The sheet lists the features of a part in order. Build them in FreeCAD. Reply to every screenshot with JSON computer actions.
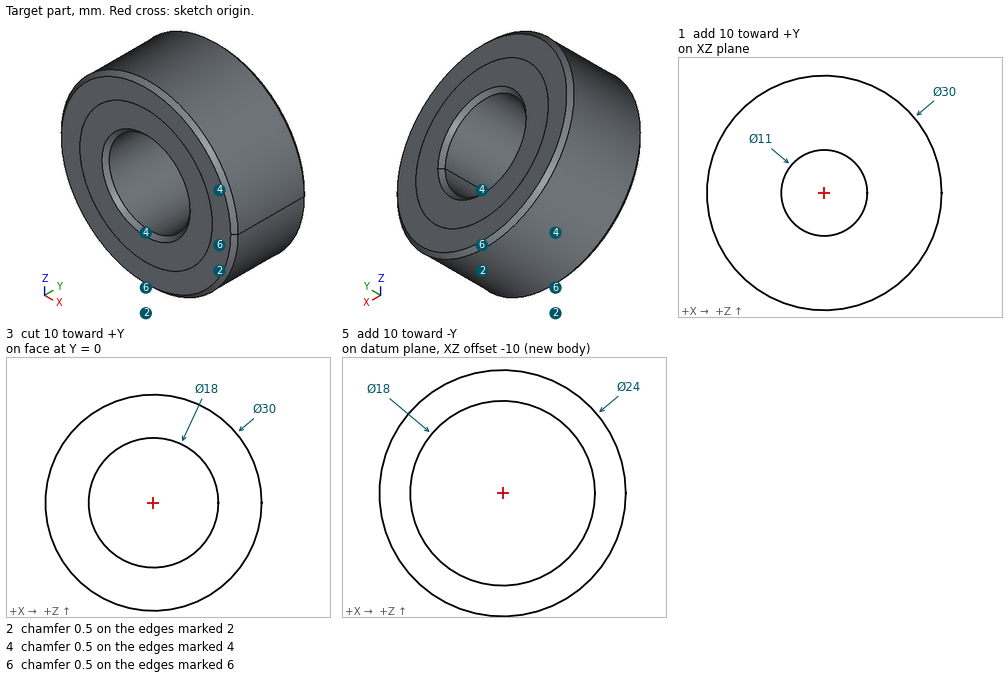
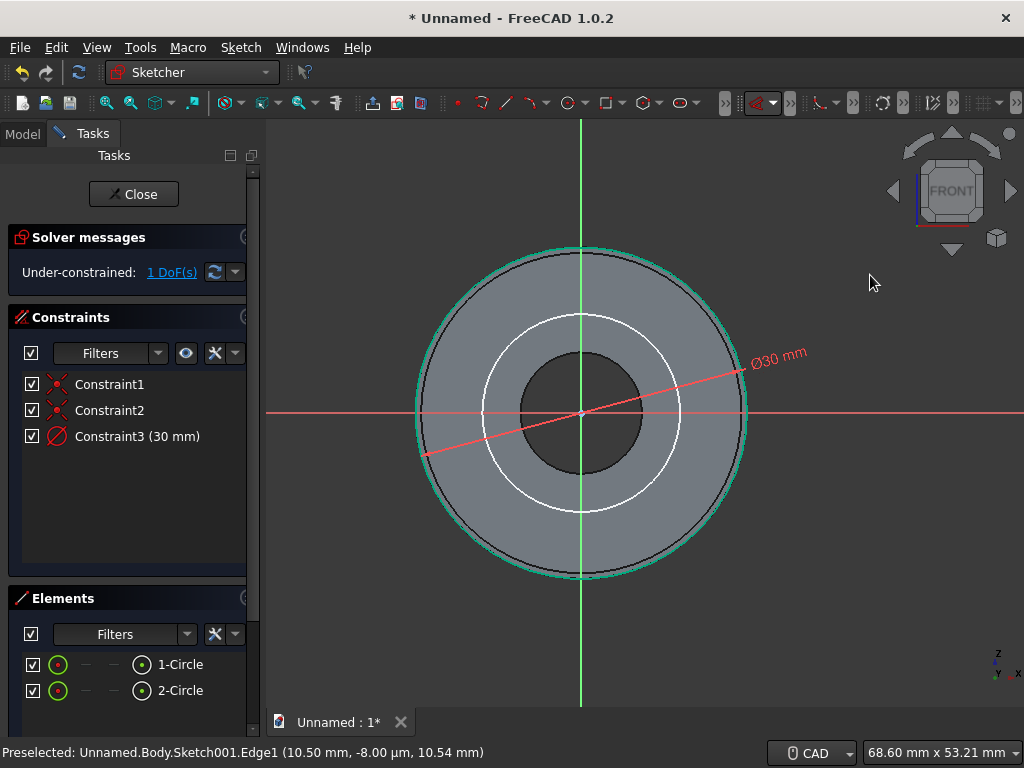
{"action": "left_click", "coordinate": [651, 343]}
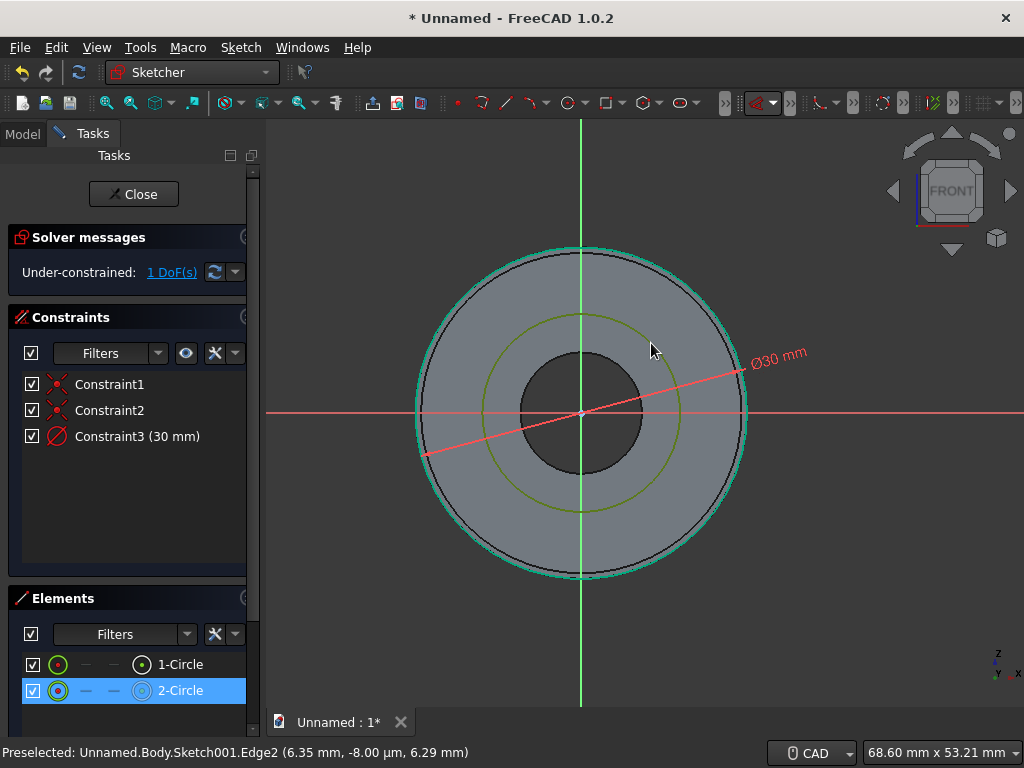
{"action": "key", "text": "k o"}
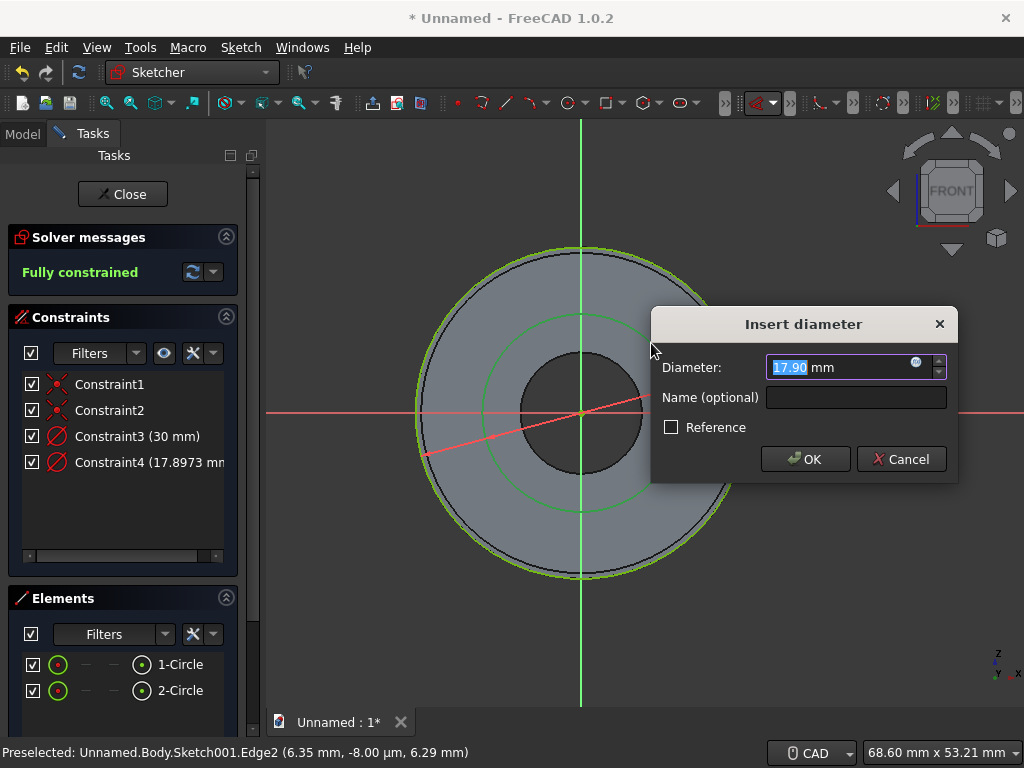
{"action": "type", "text": "18"}
{"action": "key", "text": "Return"}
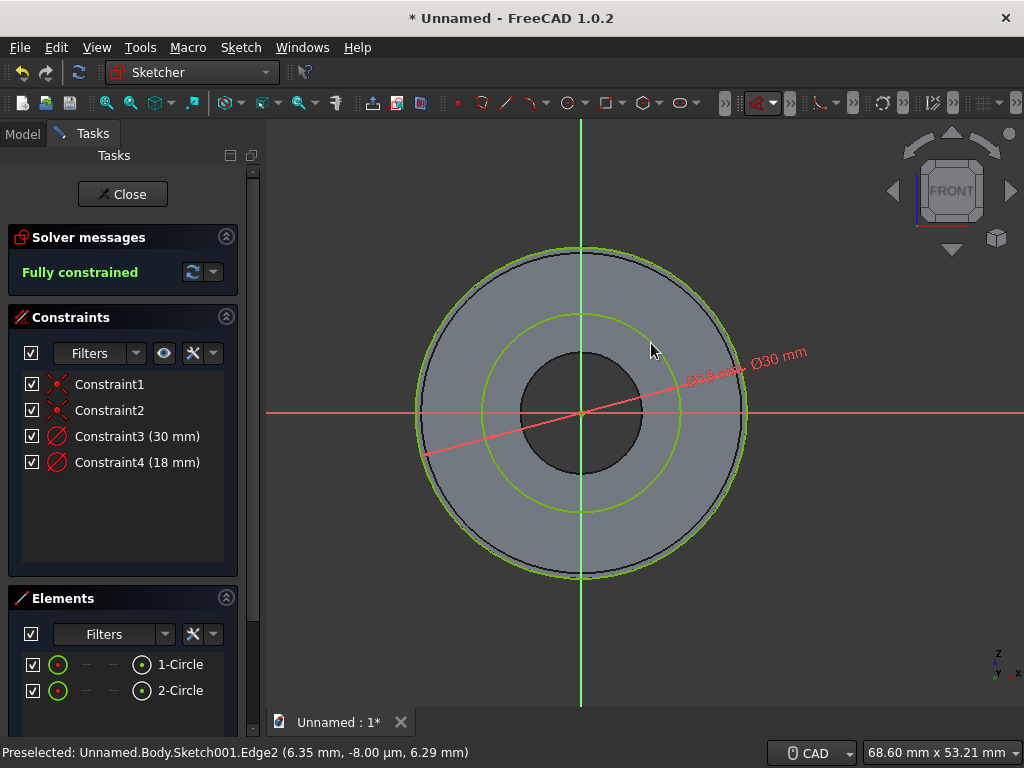
{"action": "left_click", "coordinate": [123, 194]}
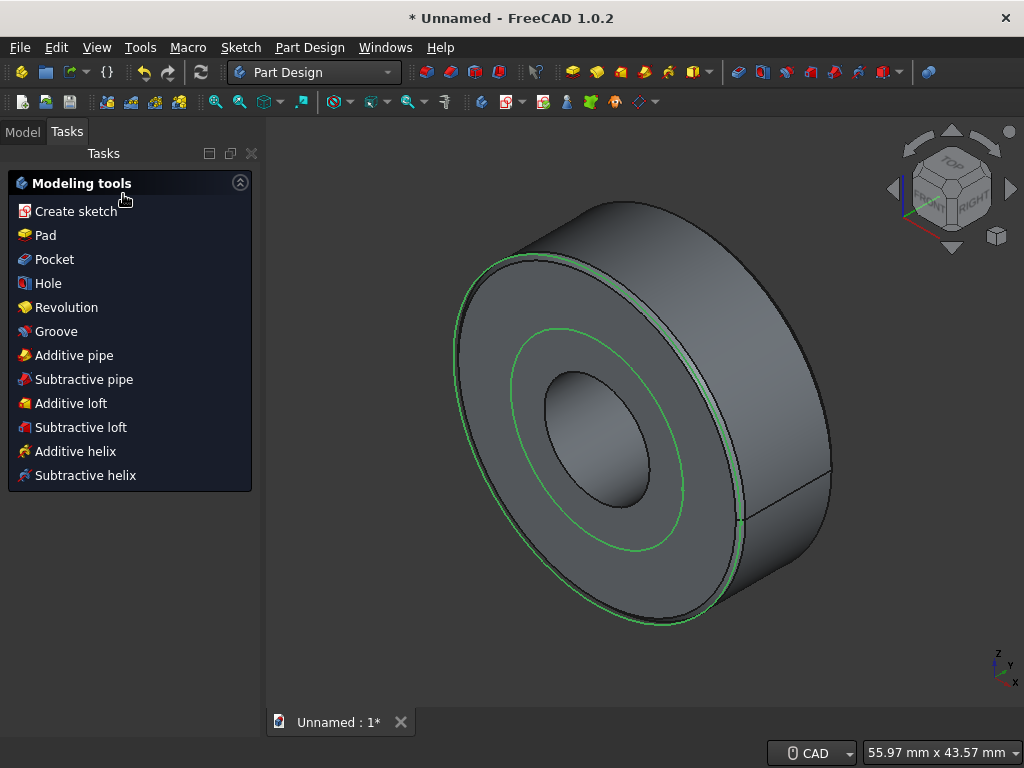
{"action": "left_click", "coordinate": [740, 72]}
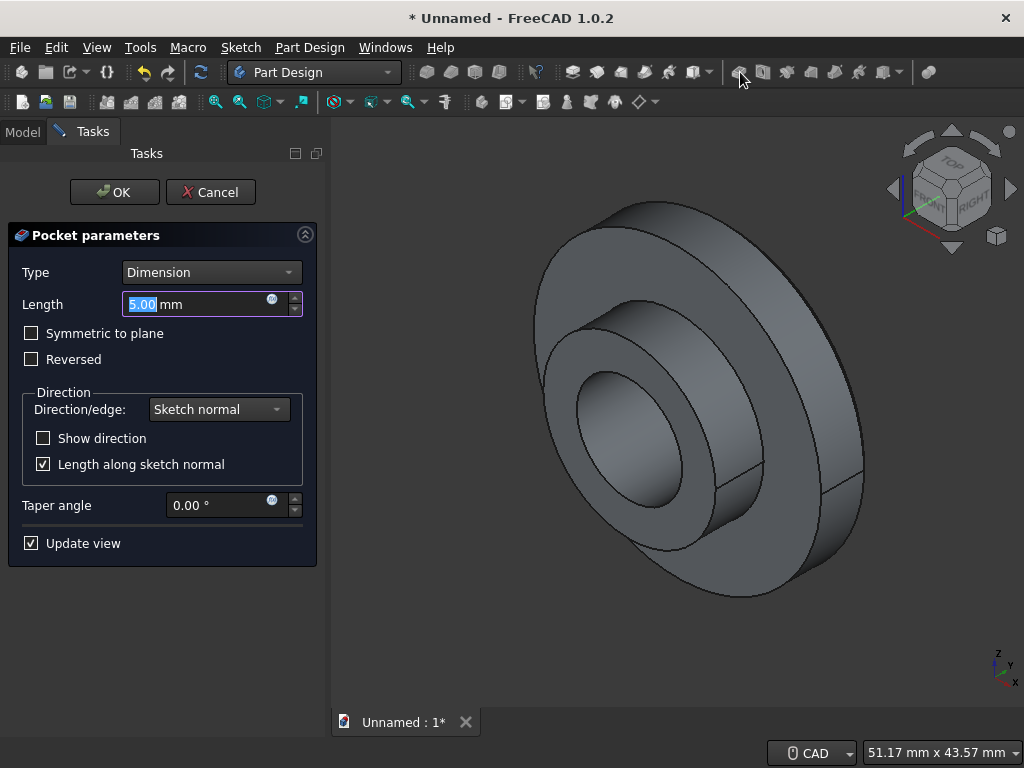
{"action": "type", "text": "10"}
{"action": "key", "text": "Tab"}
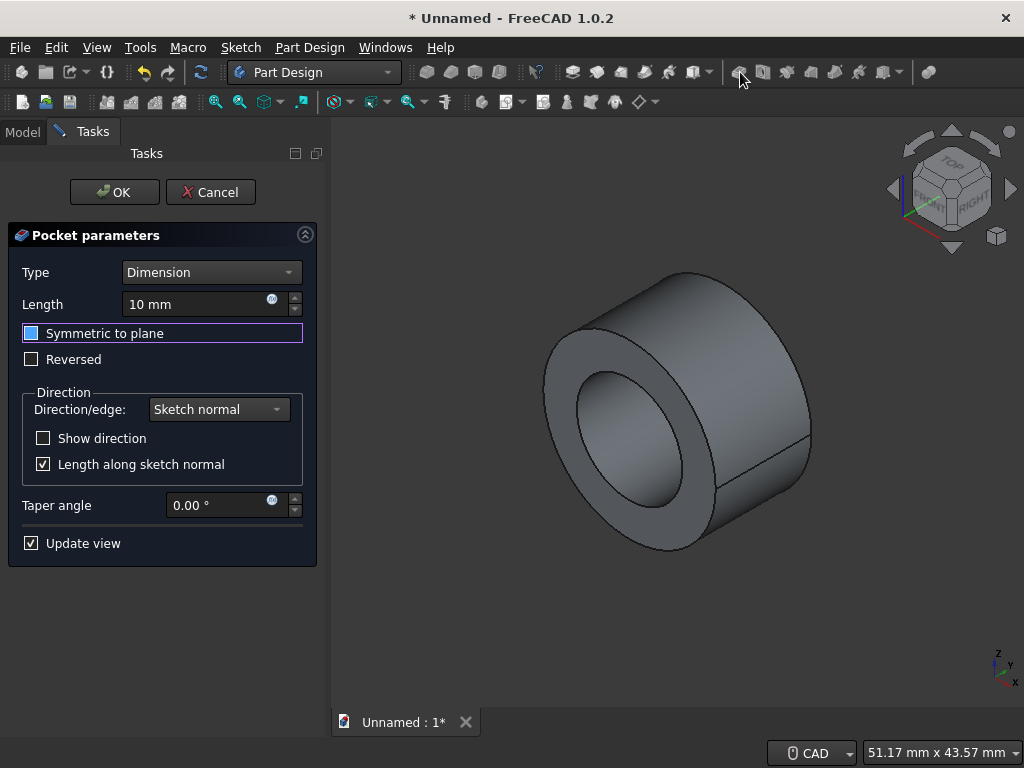
{"action": "left_click", "coordinate": [115, 192]}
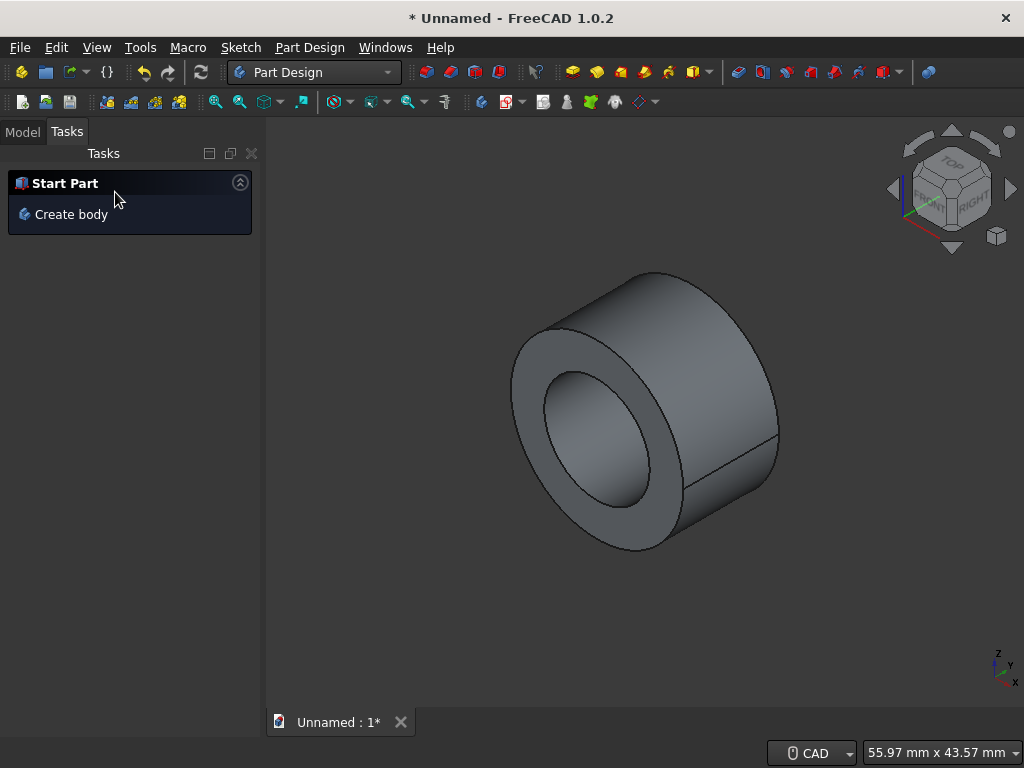
{"action": "left_click", "coordinate": [544, 408]}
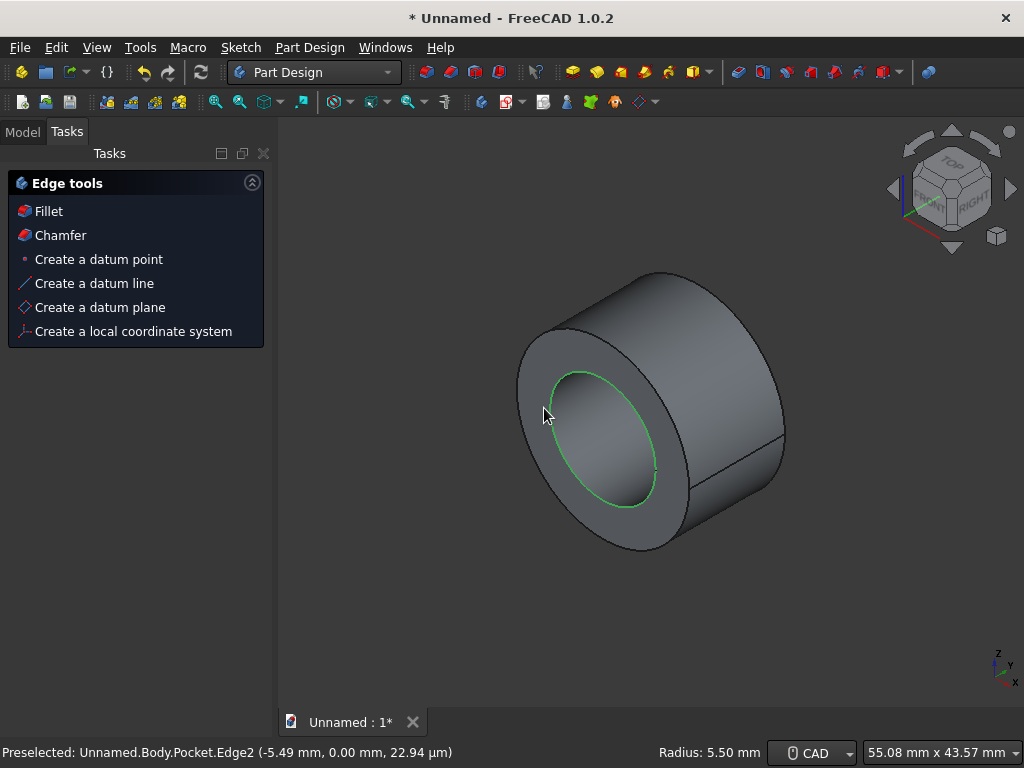
{"action": "key", "text": "2"}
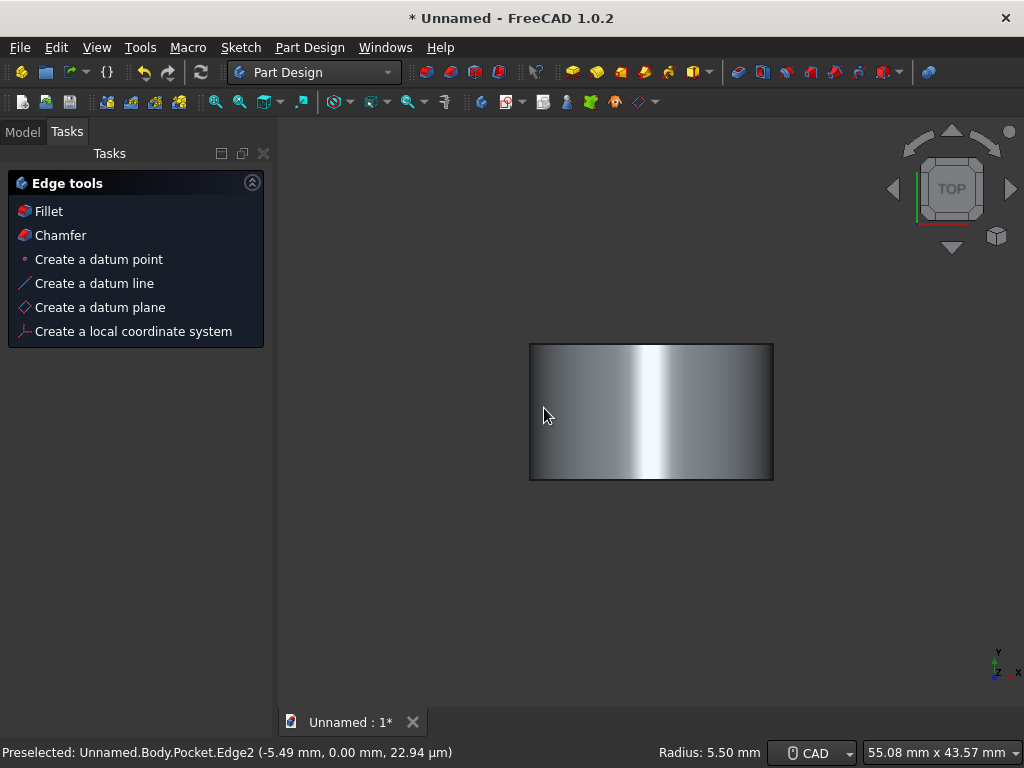
{"action": "left_click", "coordinate": [216, 102]}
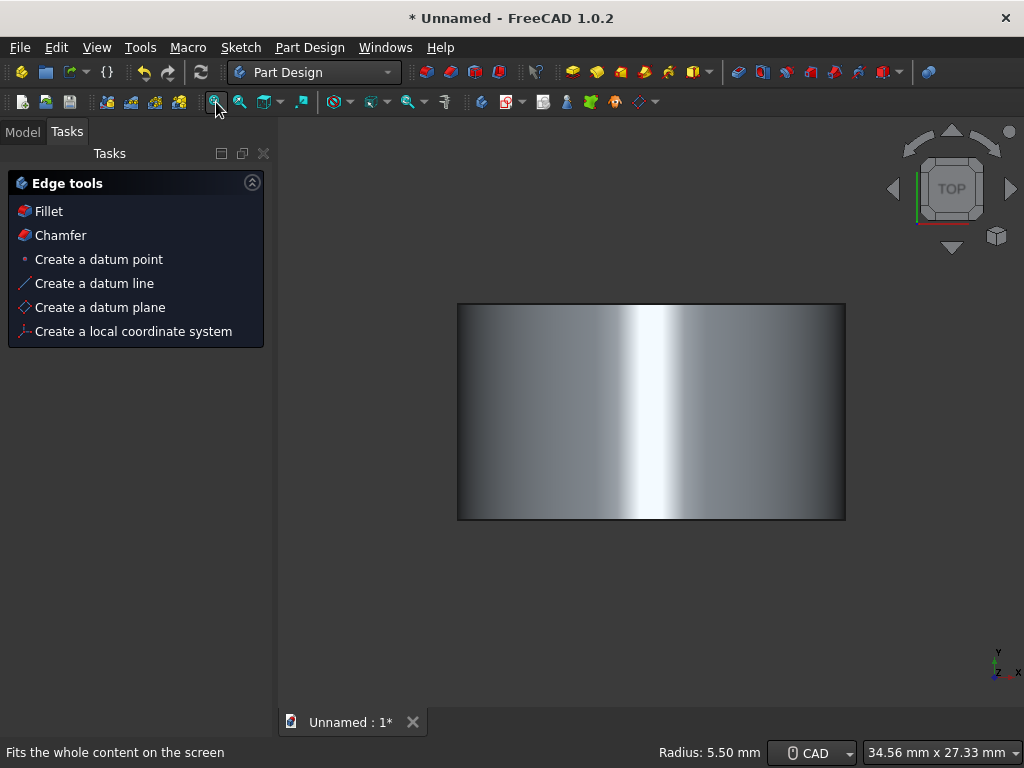
{"action": "key", "text": "0"}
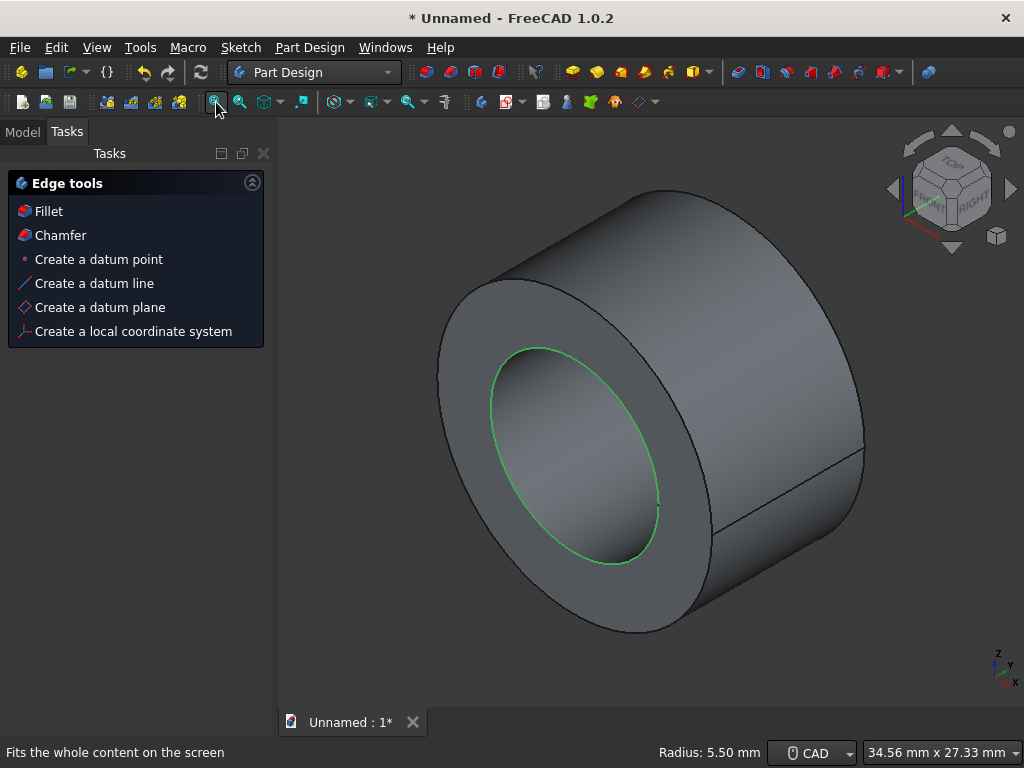
{"action": "key", "text": "1"}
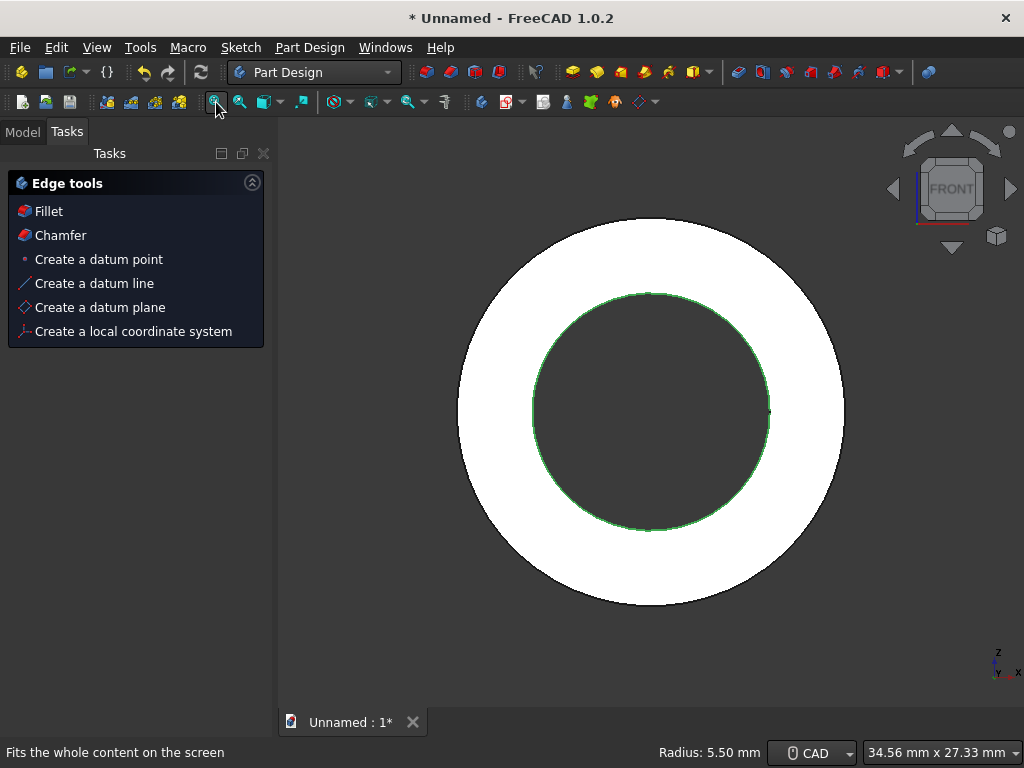
{"action": "key", "text": "3"}